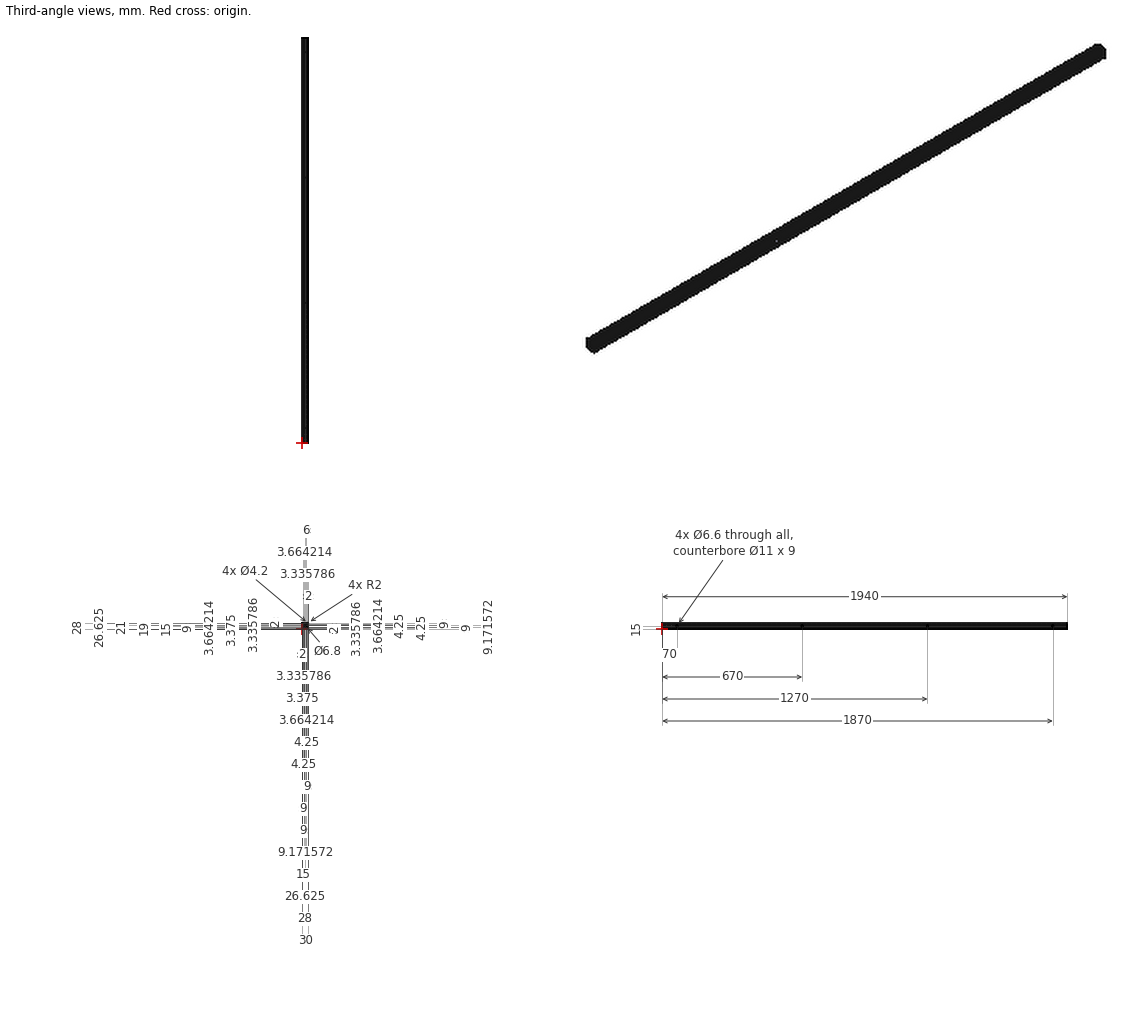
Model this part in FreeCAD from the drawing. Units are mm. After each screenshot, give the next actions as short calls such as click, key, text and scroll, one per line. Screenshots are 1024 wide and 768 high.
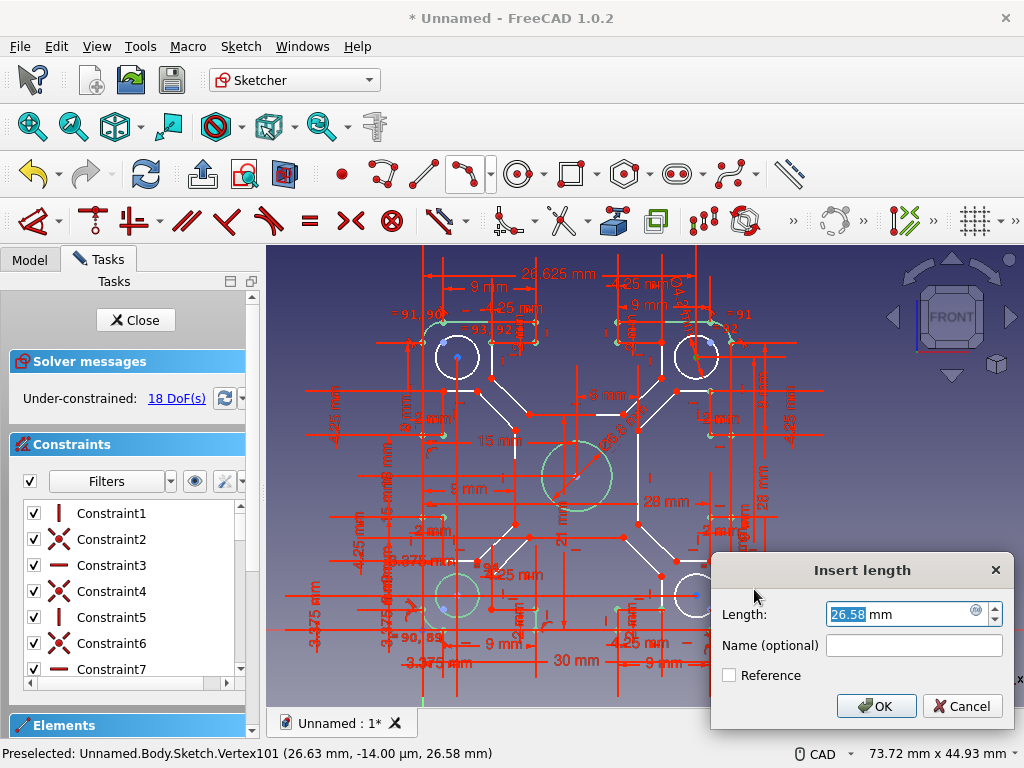
text(26.625)
key(Return)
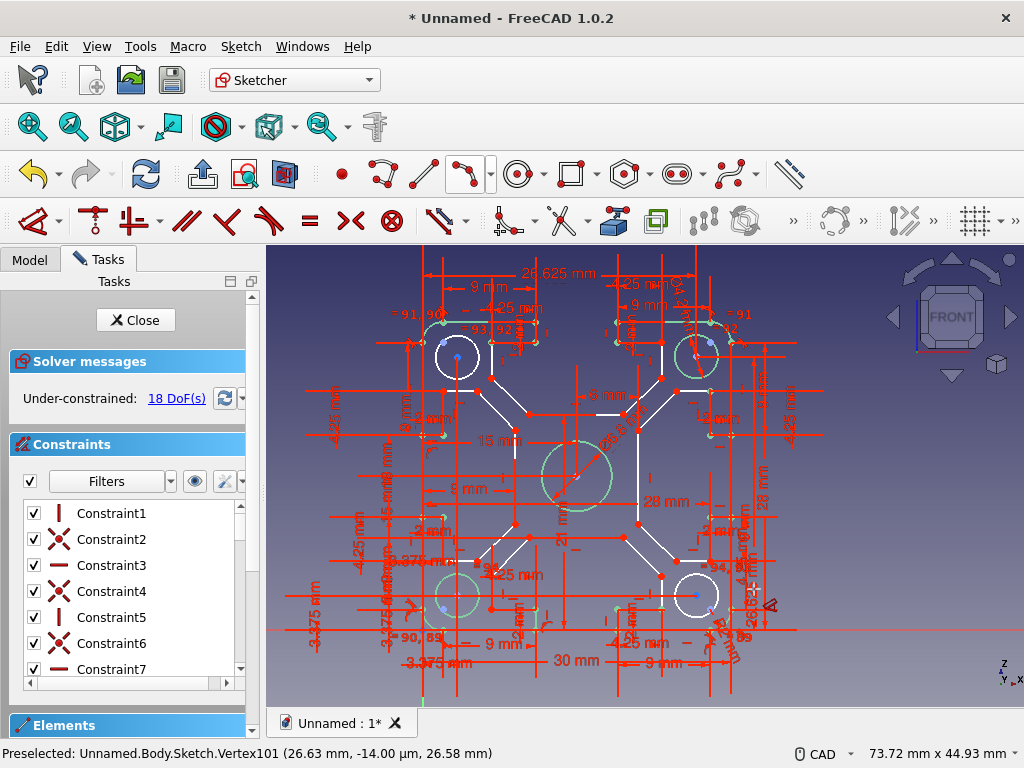
click(457, 357)
click(317, 494)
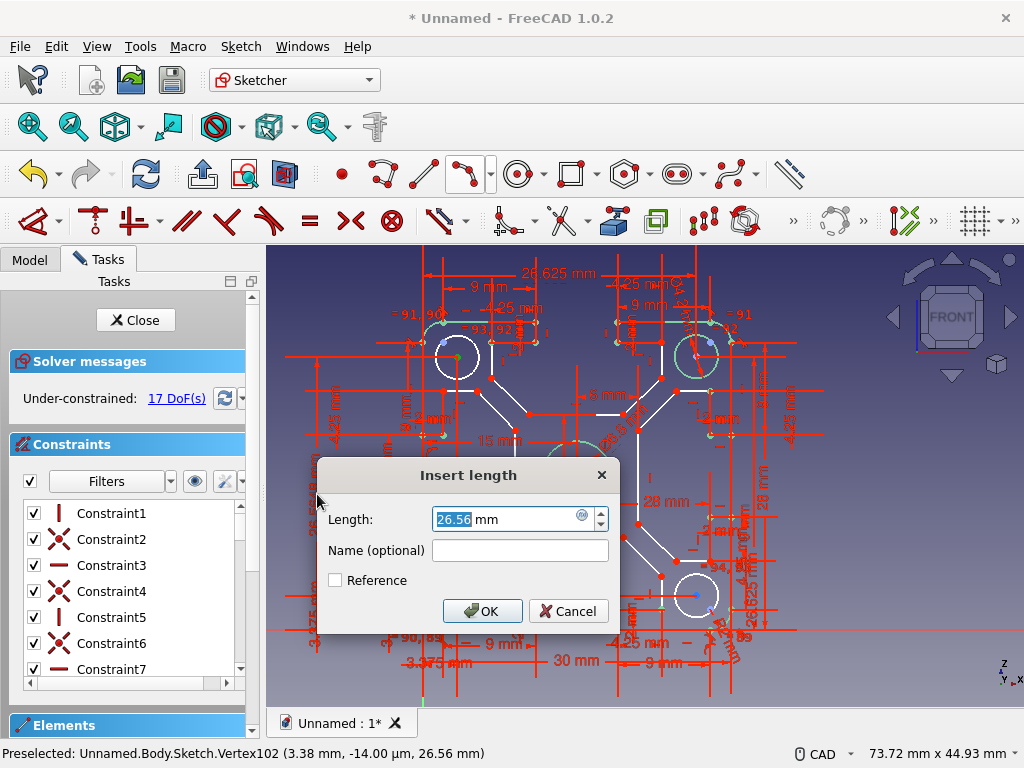
text(26.625)
key(Return)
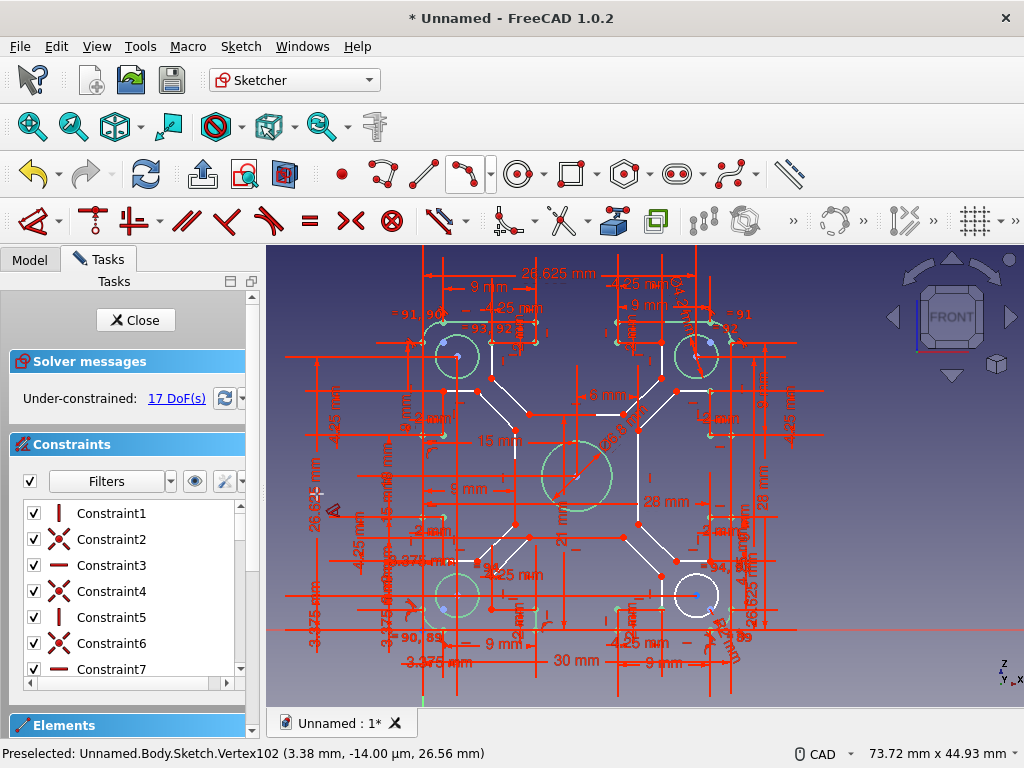
click(697, 596)
click(623, 562)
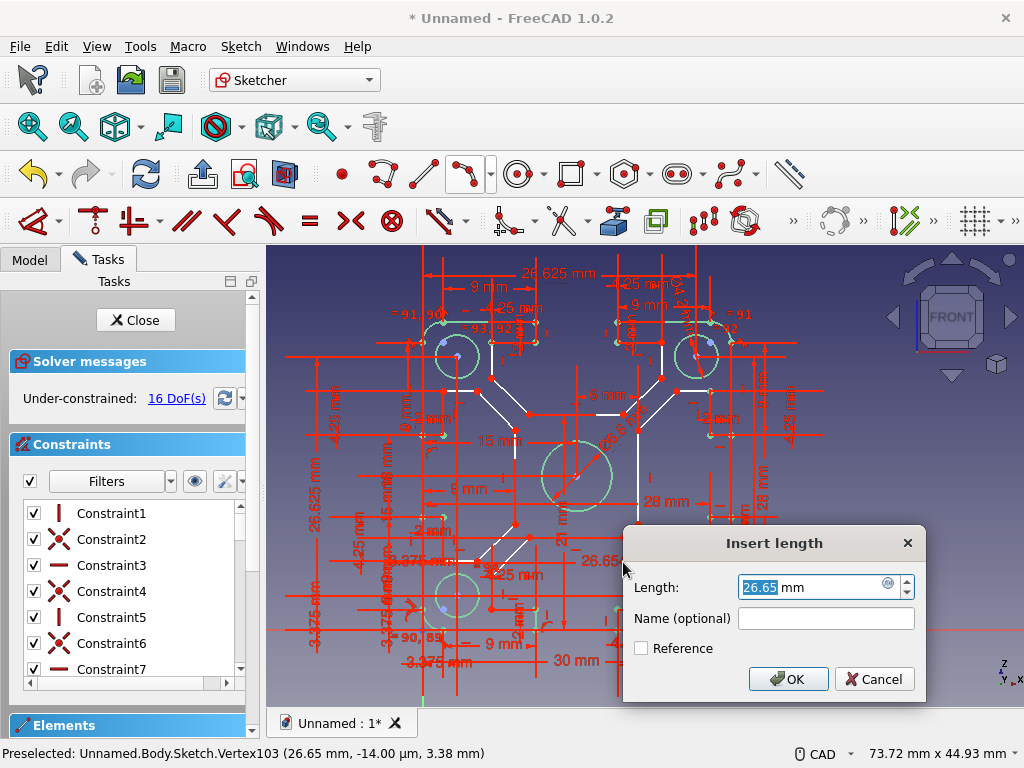
text(26.625)
key(Return)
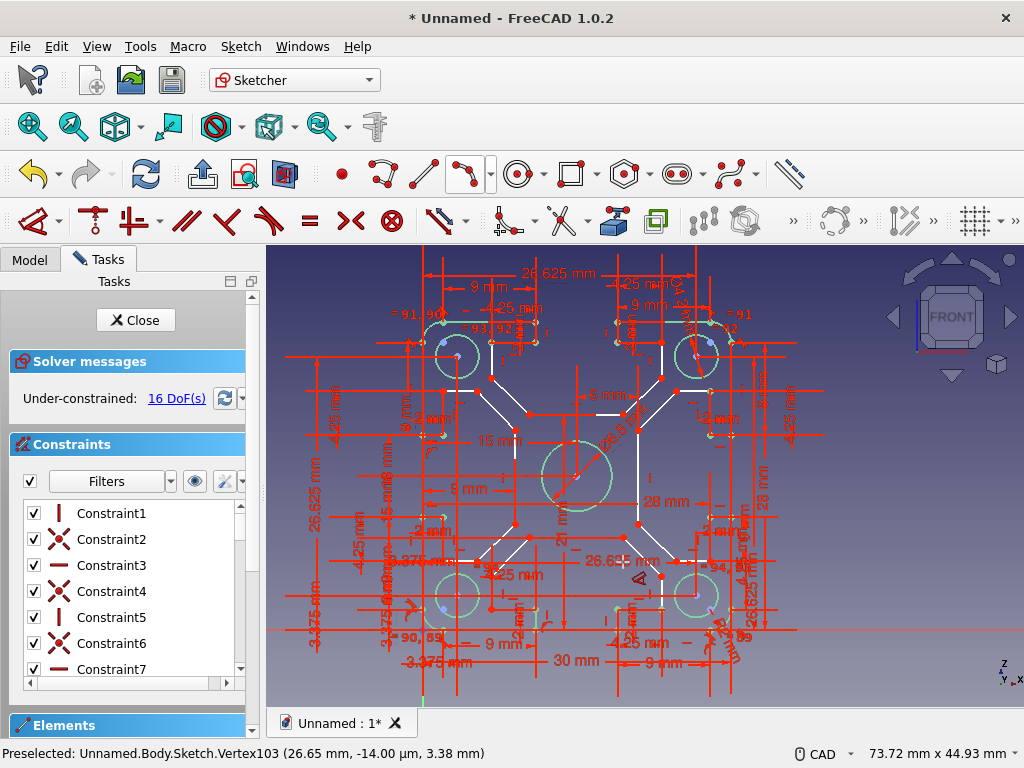
scroll(700, 391, up, 2)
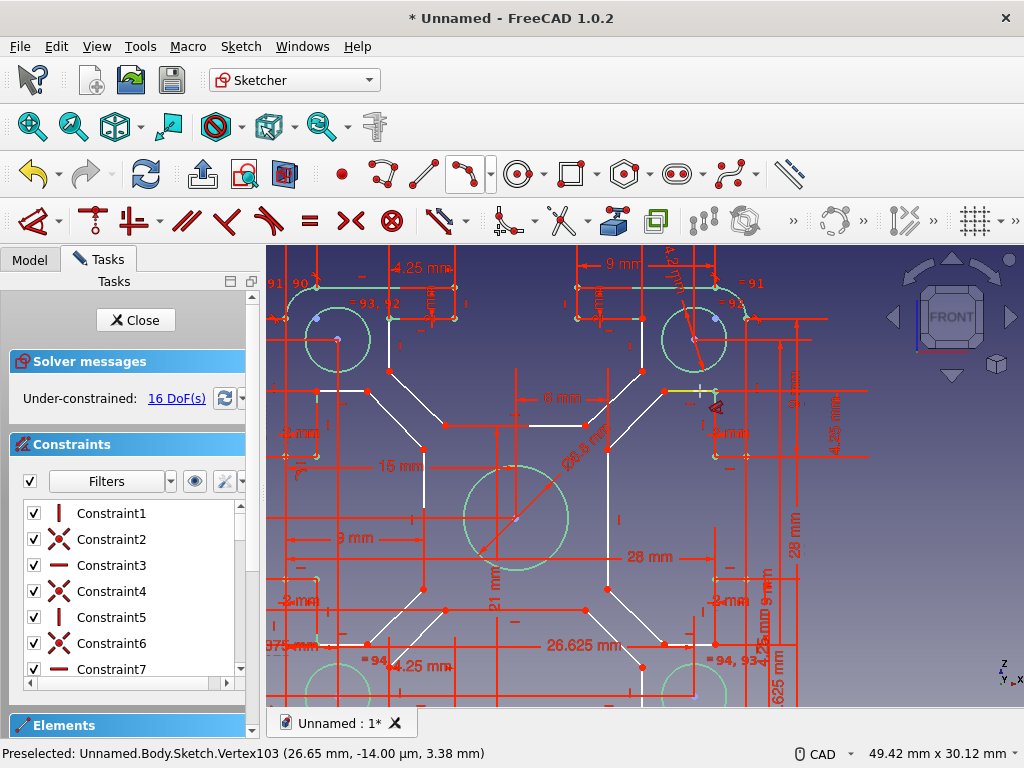
click(700, 391)
click(690, 357)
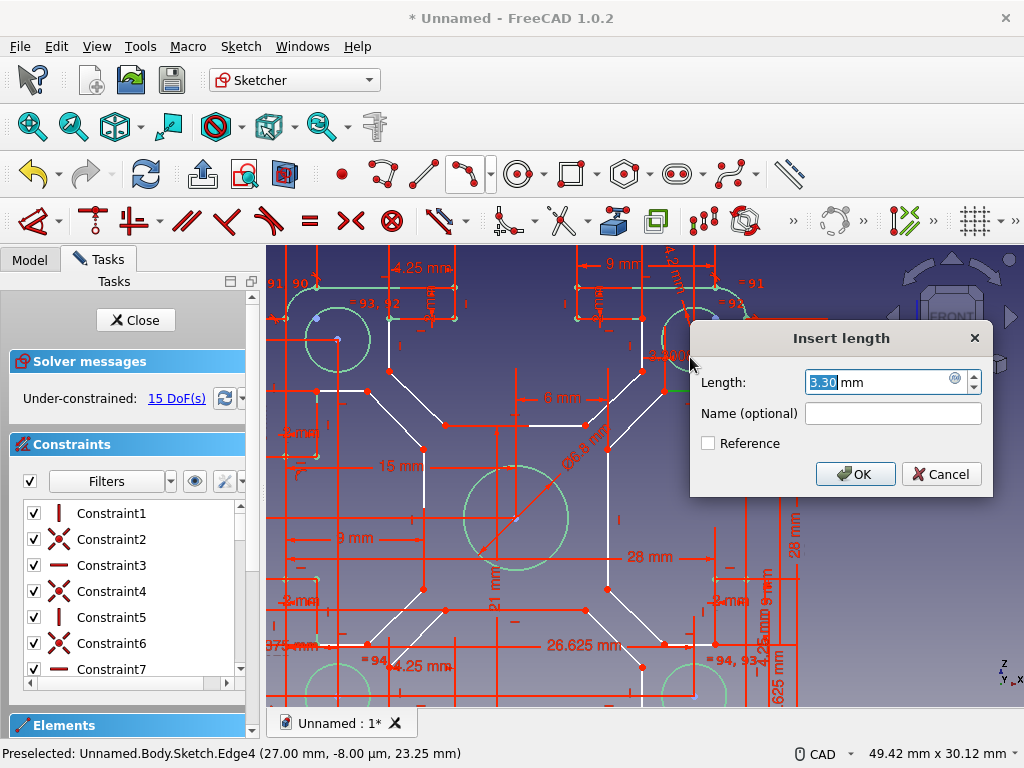
text(3.335786)
key(Return)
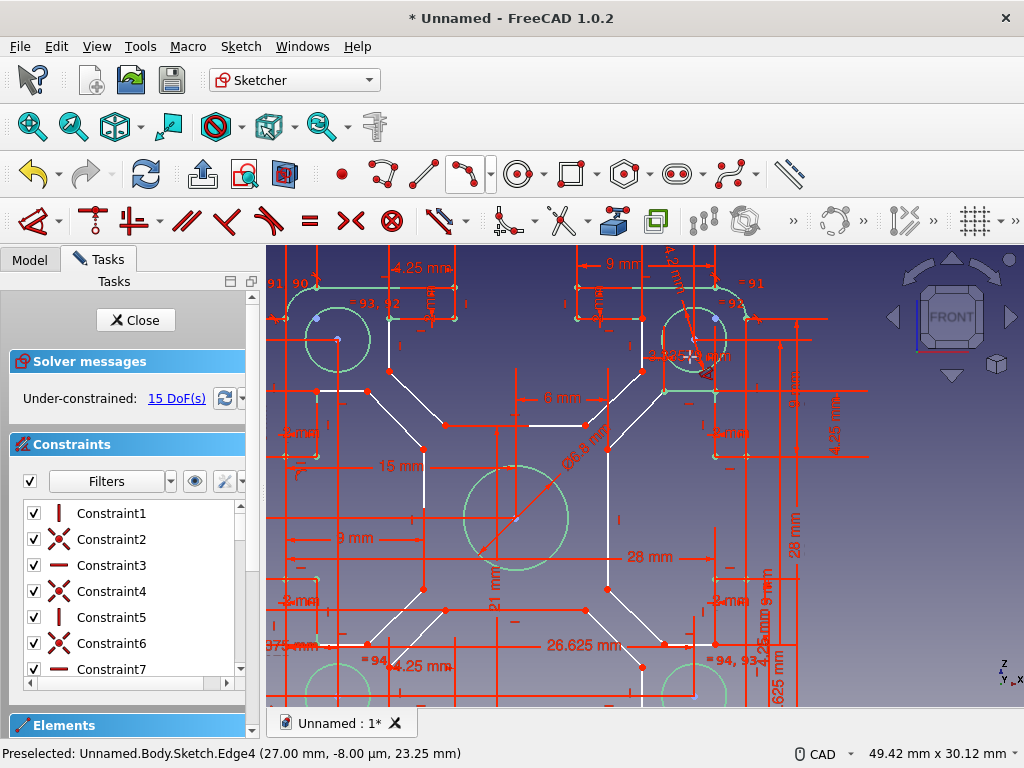
click(608, 492)
click(642, 520)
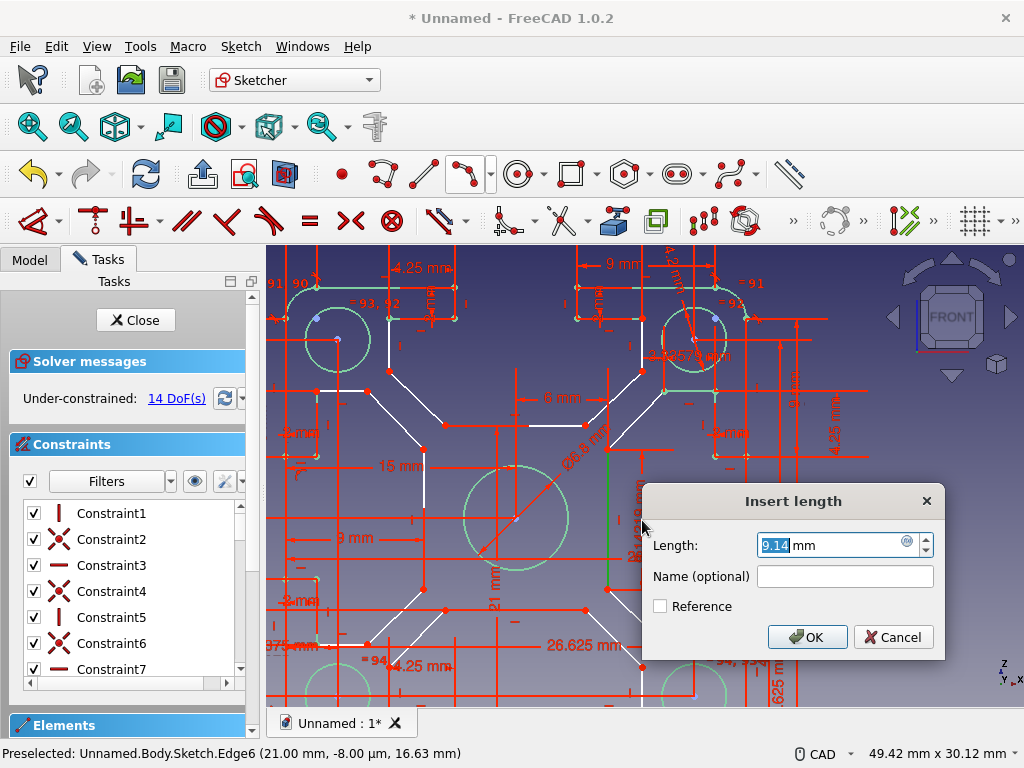
text(9.171572)
key(Return)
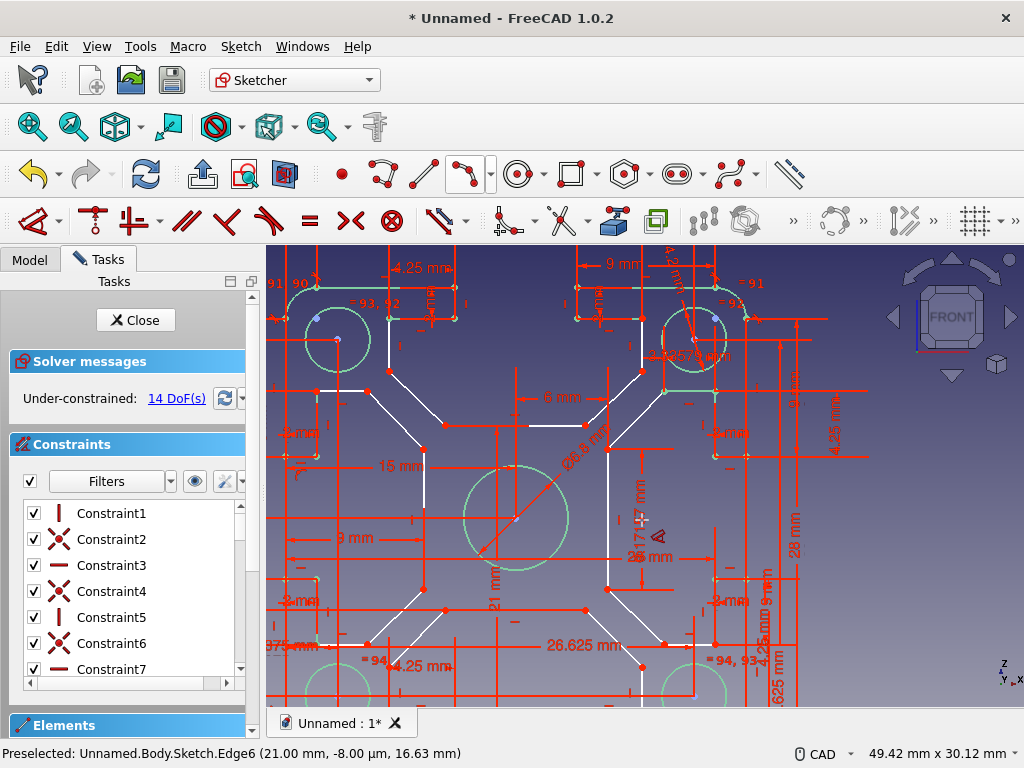
click(680, 645)
click(690, 679)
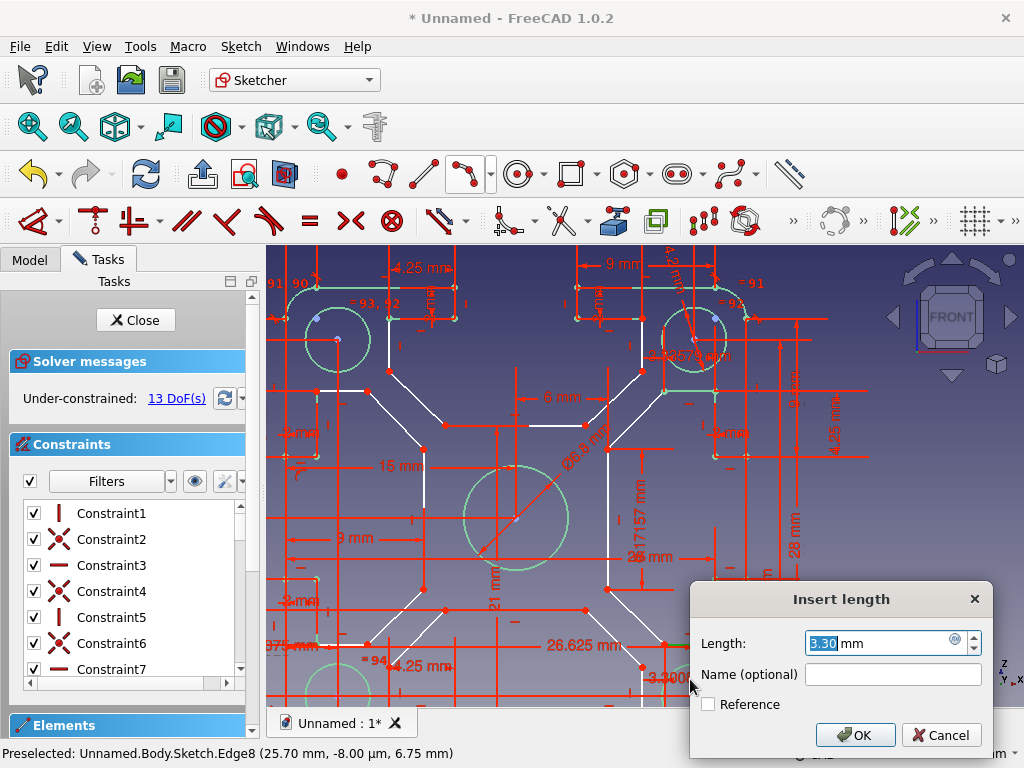
text(3.335786)
key(Return)